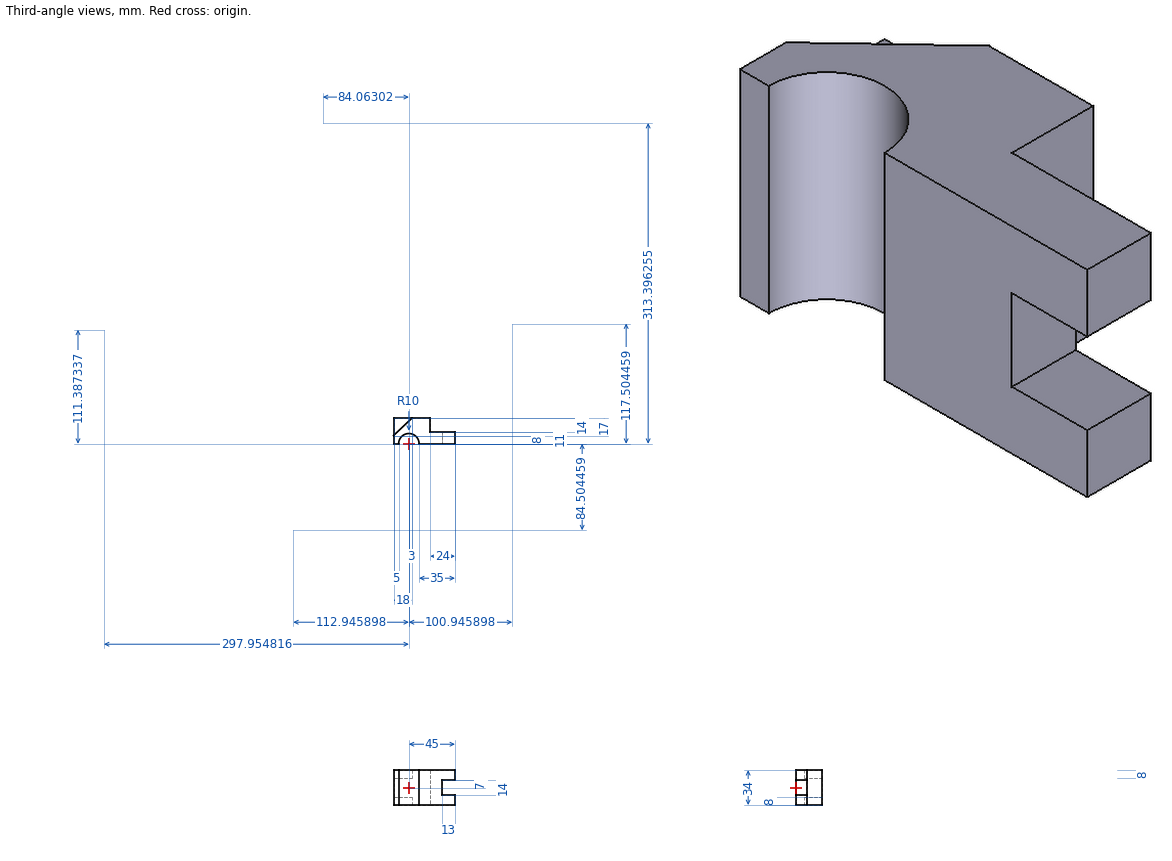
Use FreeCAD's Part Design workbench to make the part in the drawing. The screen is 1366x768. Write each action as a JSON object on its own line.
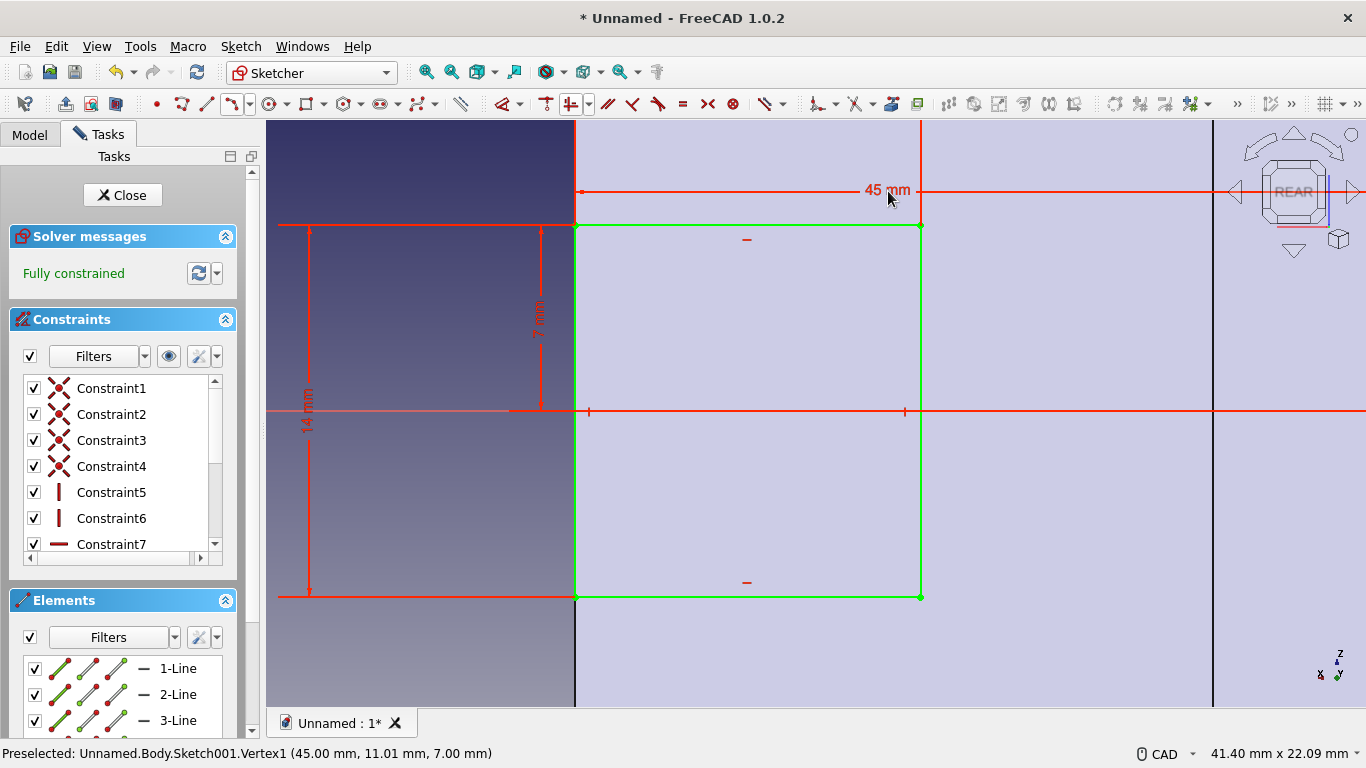
{"action": "left_click", "coordinate": [123, 195]}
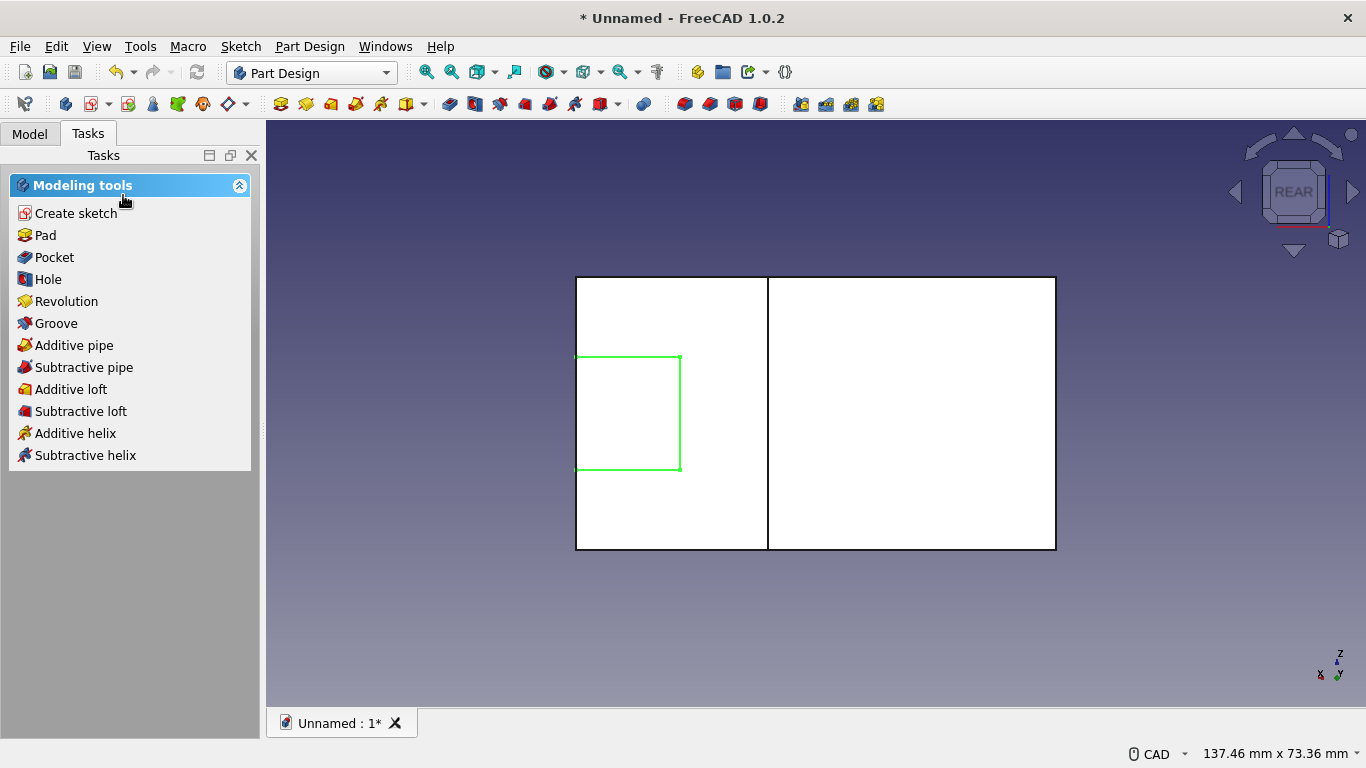
{"action": "left_click", "coordinate": [450, 104]}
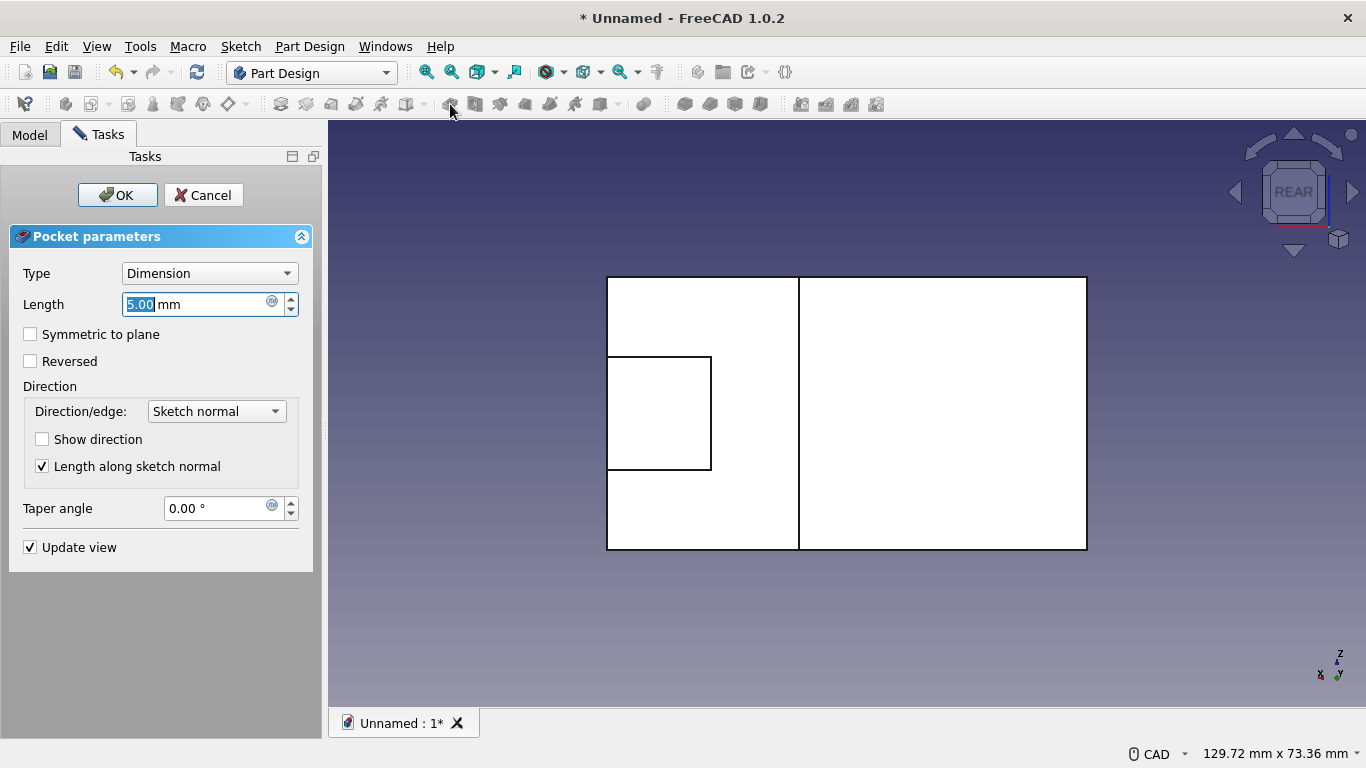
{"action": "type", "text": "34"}
{"action": "key", "text": "Tab"}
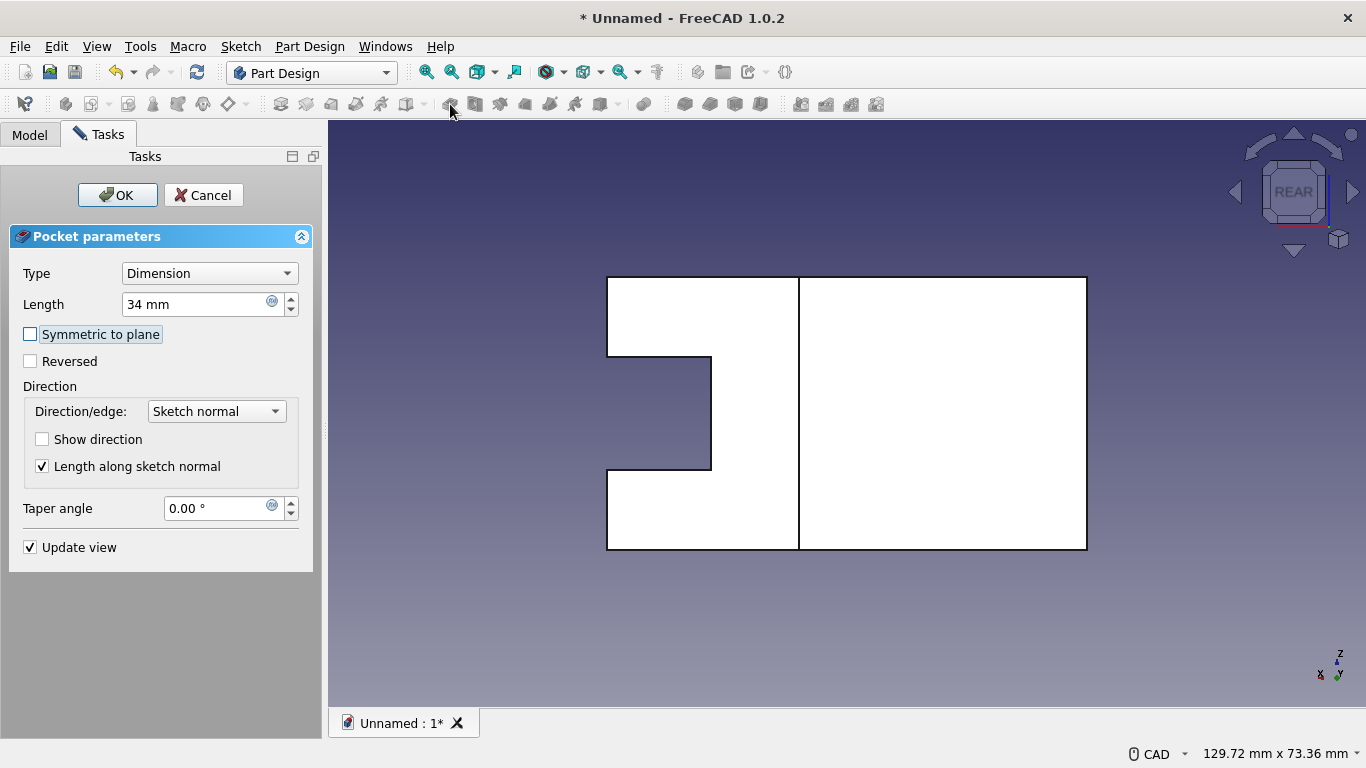
{"action": "left_click", "coordinate": [31, 334]}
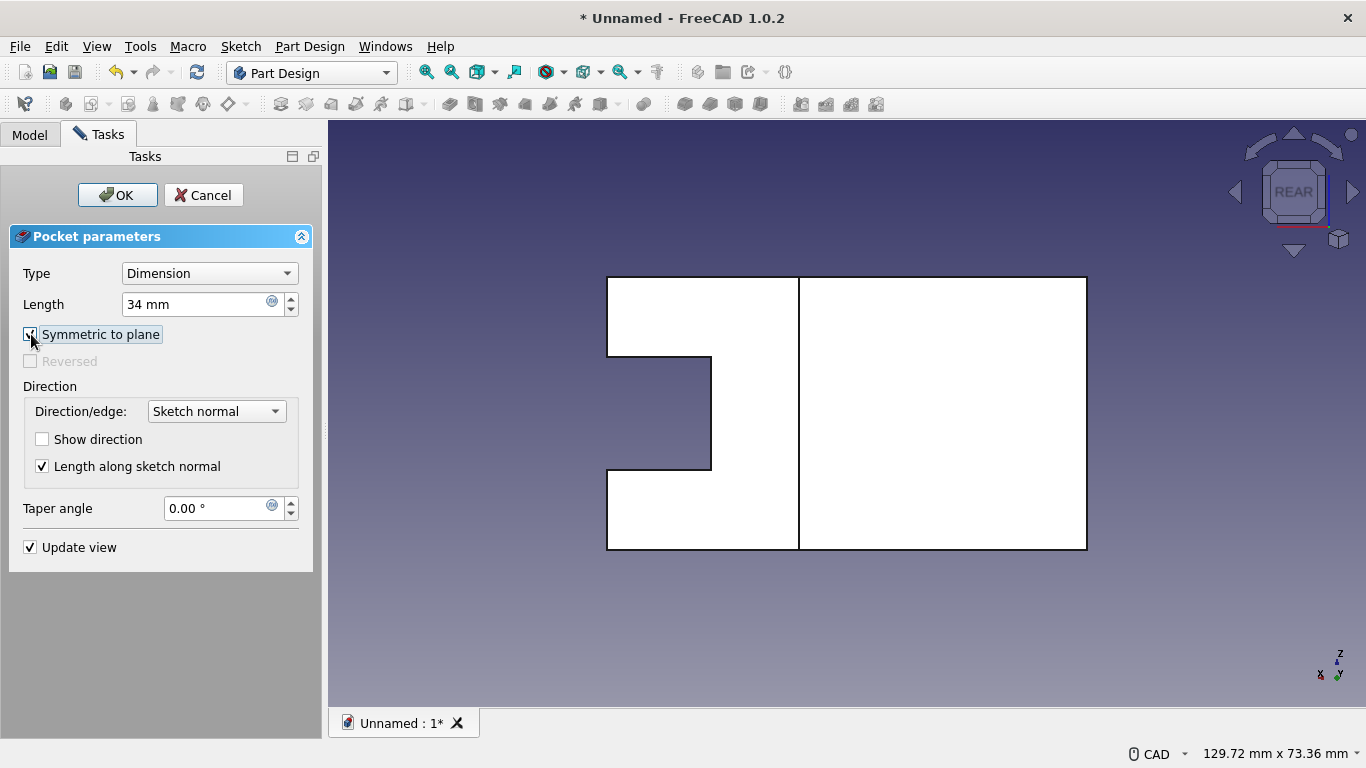
{"action": "left_click", "coordinate": [118, 195]}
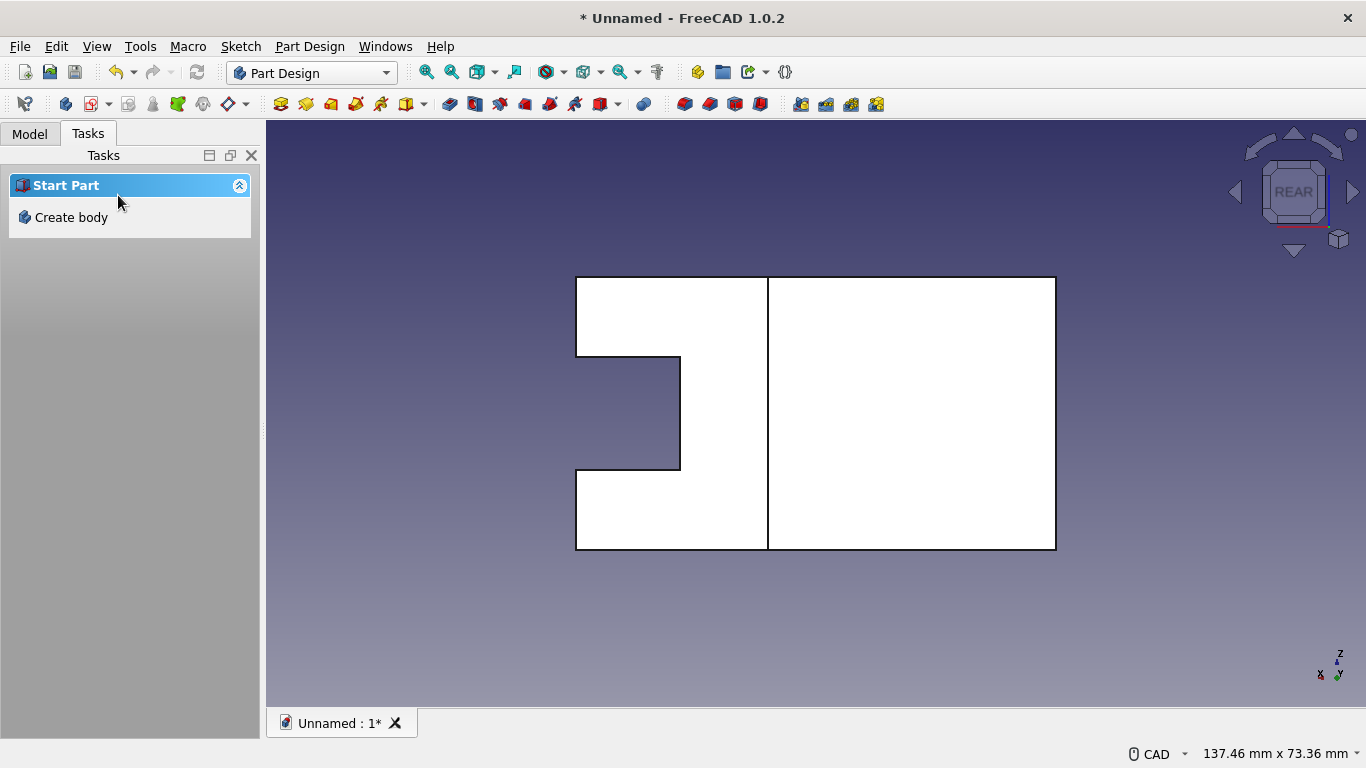
{"action": "key", "text": "0"}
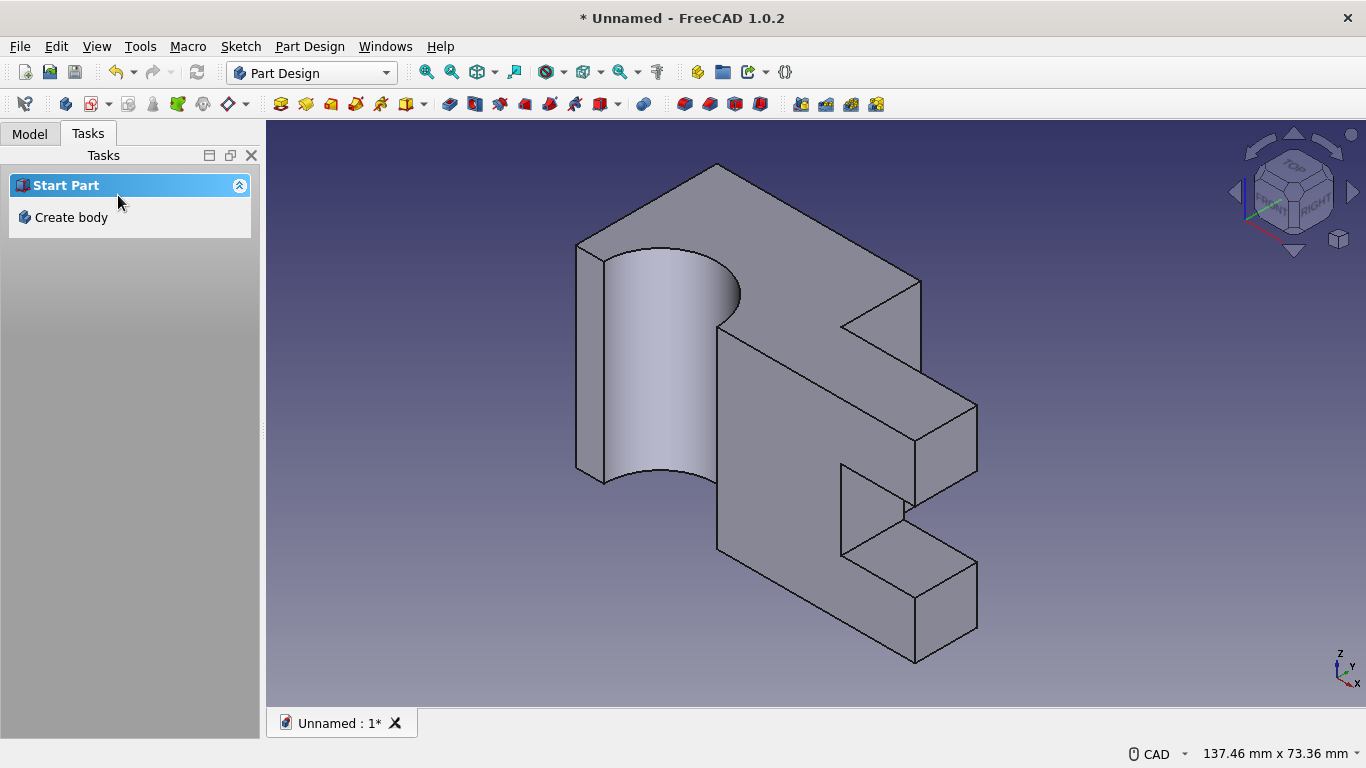
{"action": "left_click", "coordinate": [788, 262]}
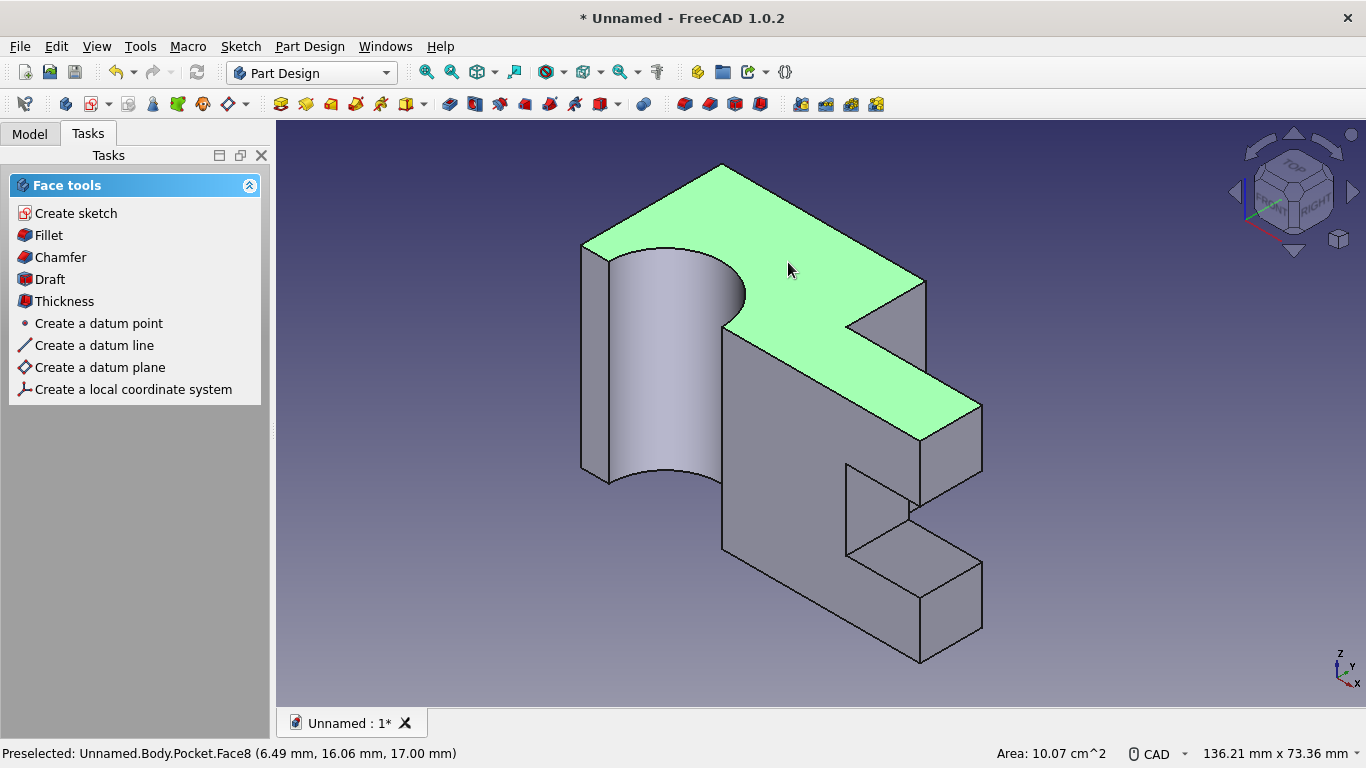
{"action": "left_click", "coordinate": [90, 104]}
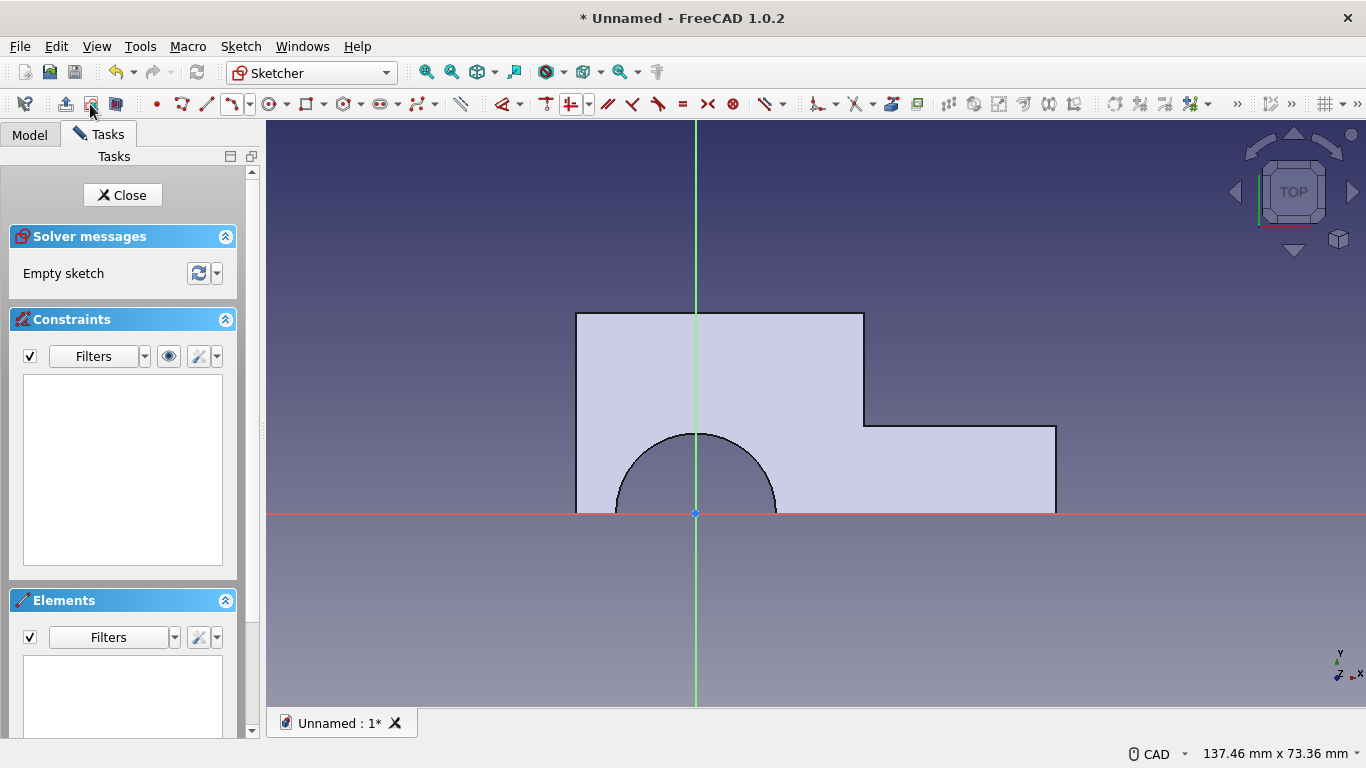
{"action": "scroll", "coordinate": [852, 515], "scroll_direction": "down", "scroll_amount": 11}